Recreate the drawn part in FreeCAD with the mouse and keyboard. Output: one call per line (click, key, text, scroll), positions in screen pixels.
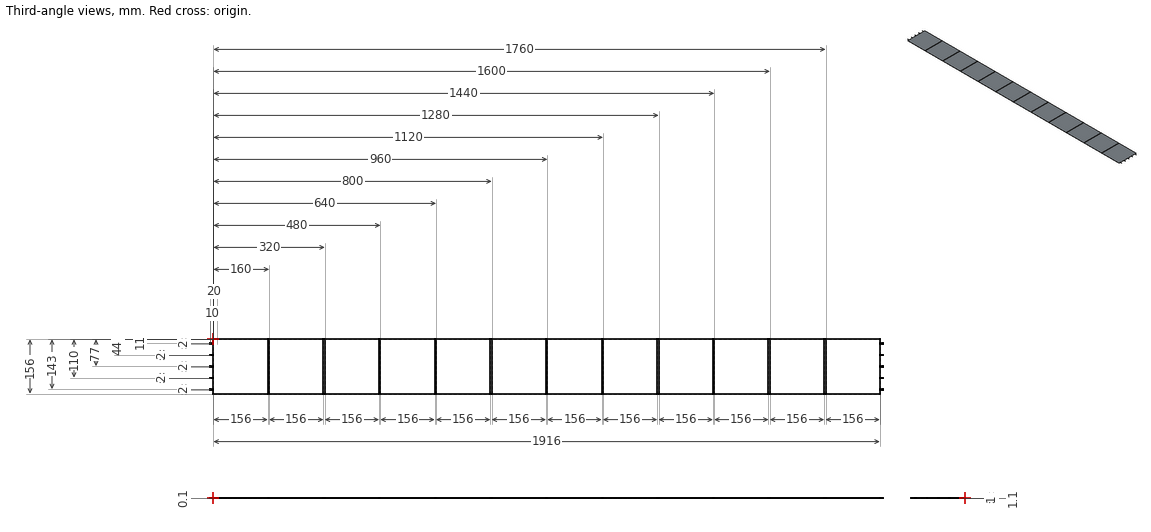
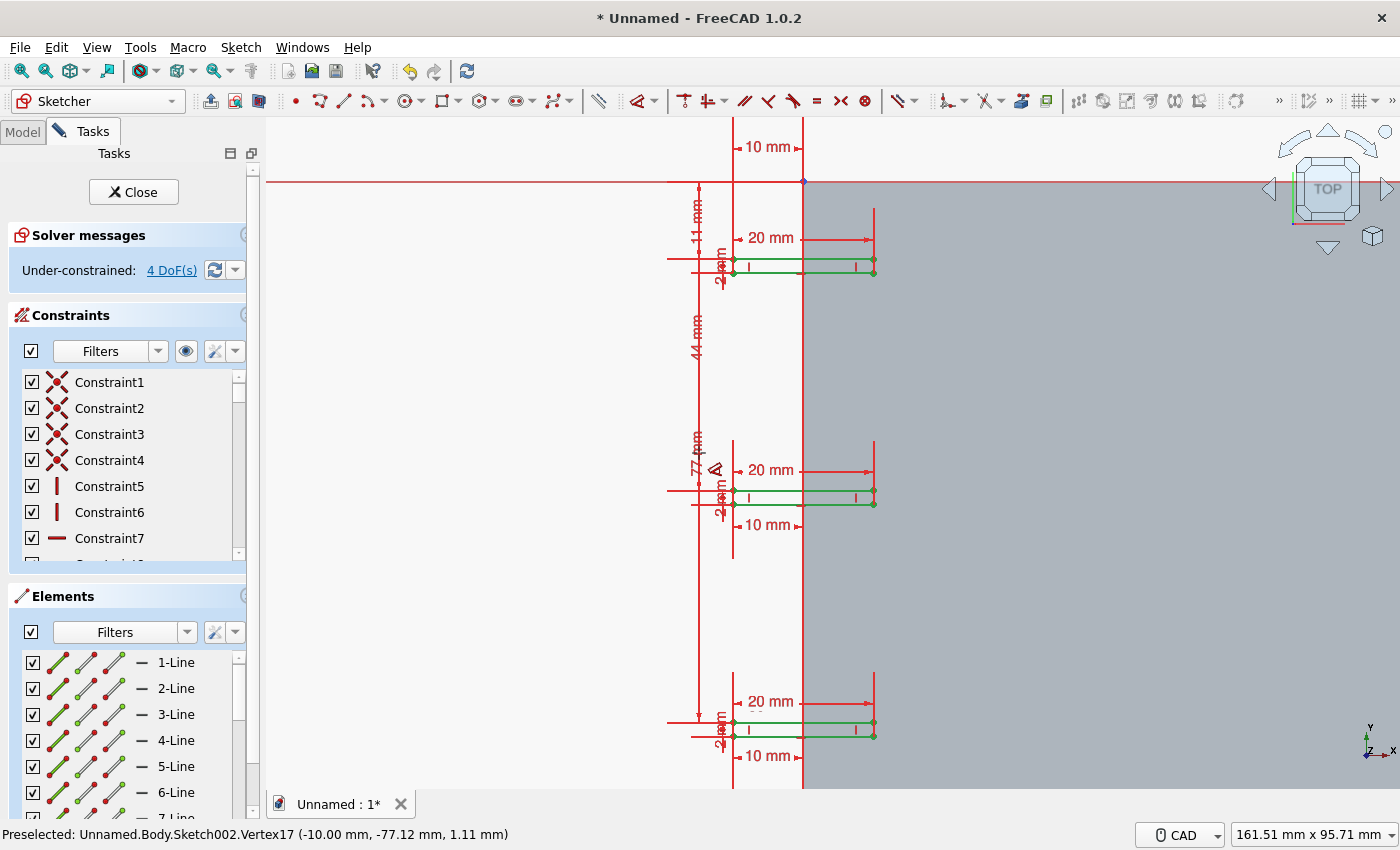
scroll(733, 259, down, 4)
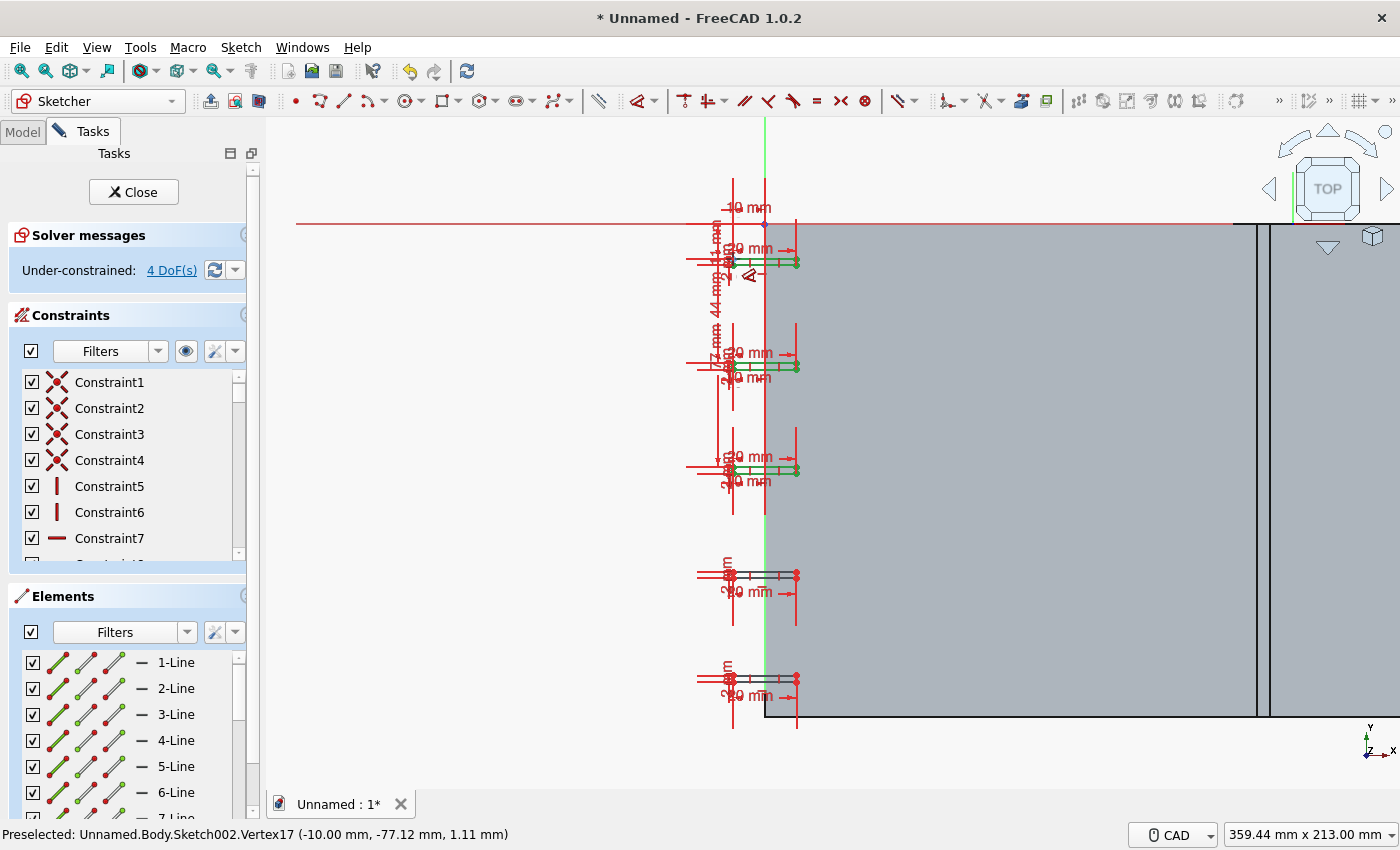
scroll(733, 572, up, 4)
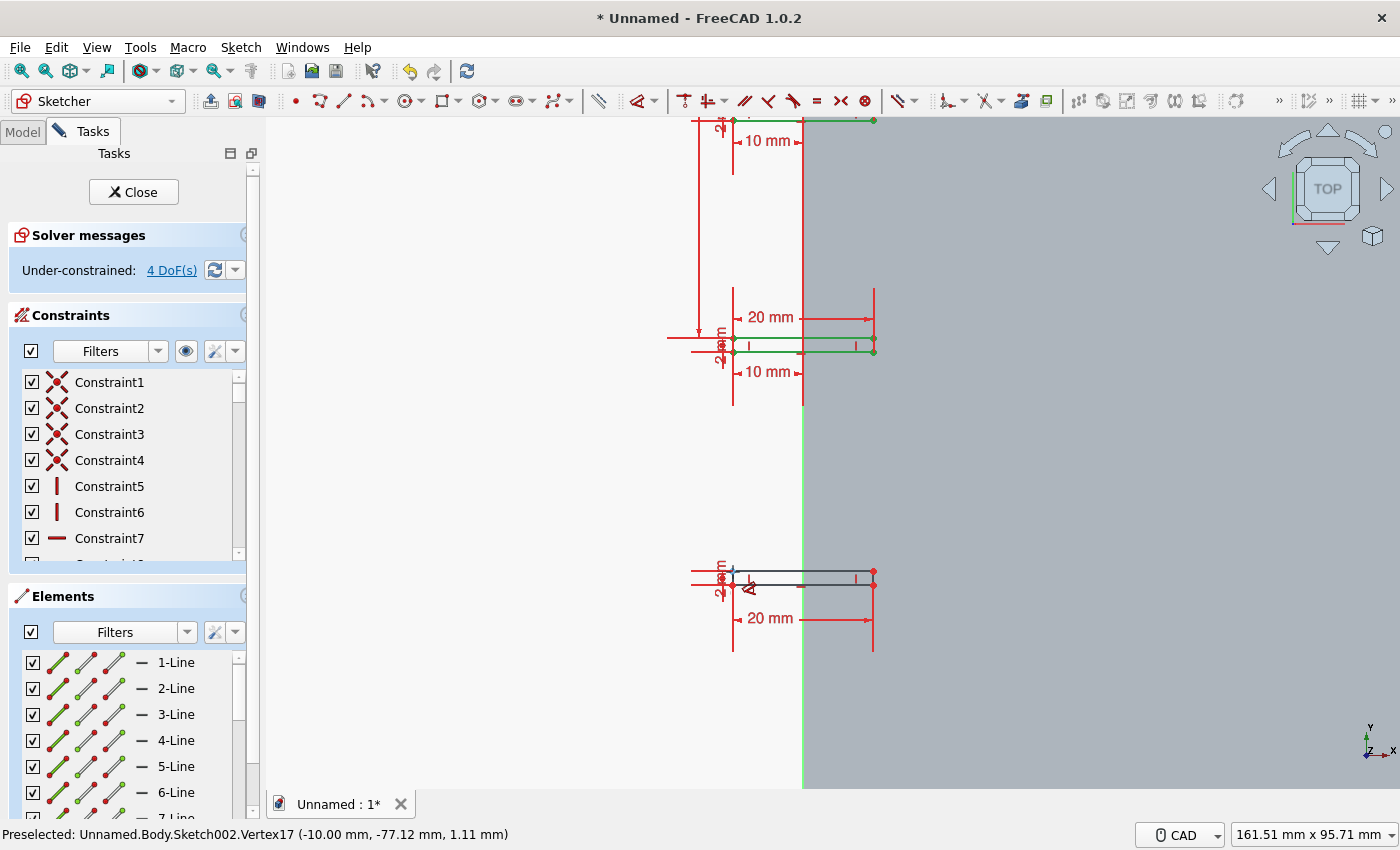
click(733, 571)
click(768, 653)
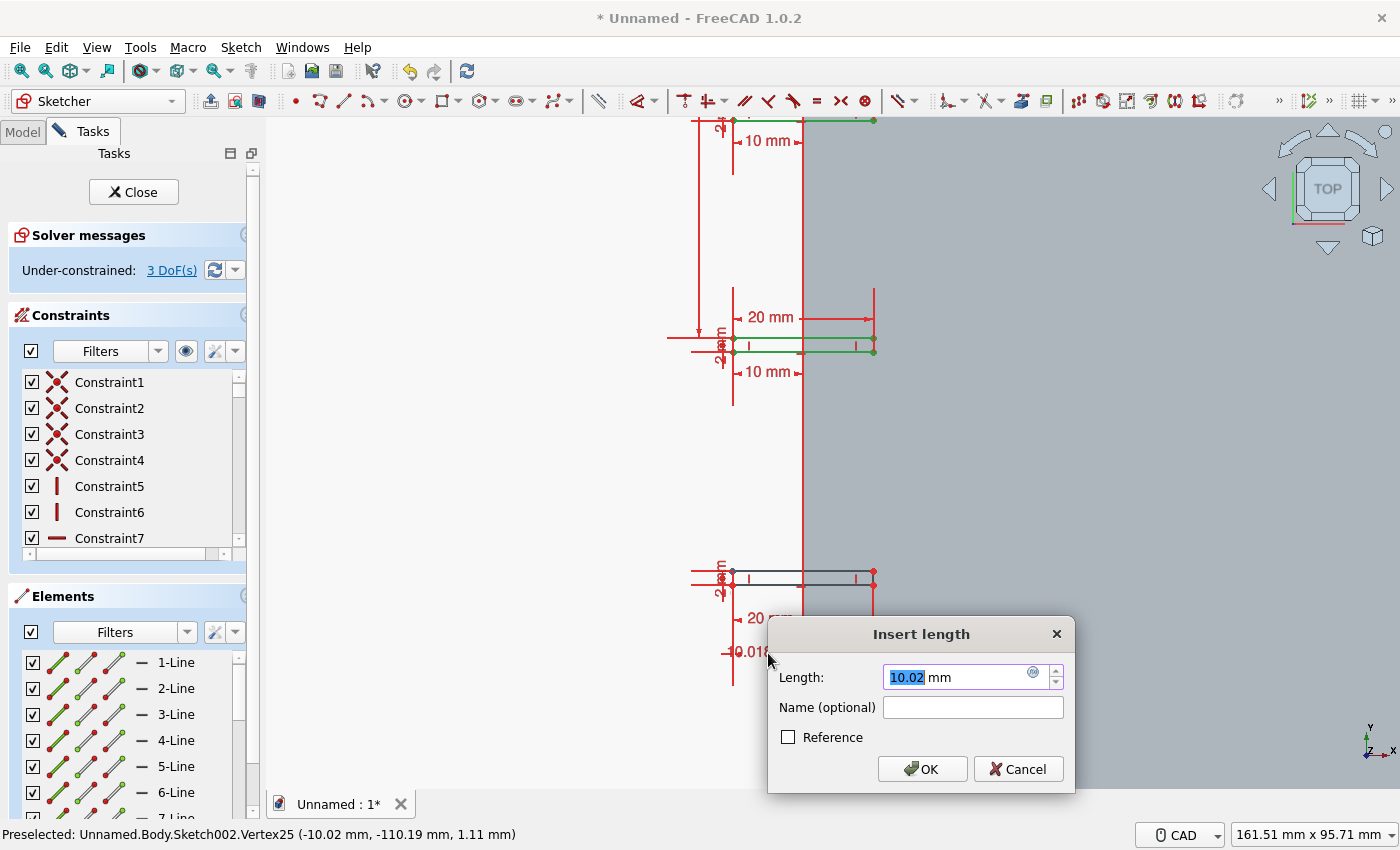
text(10)
key(Return)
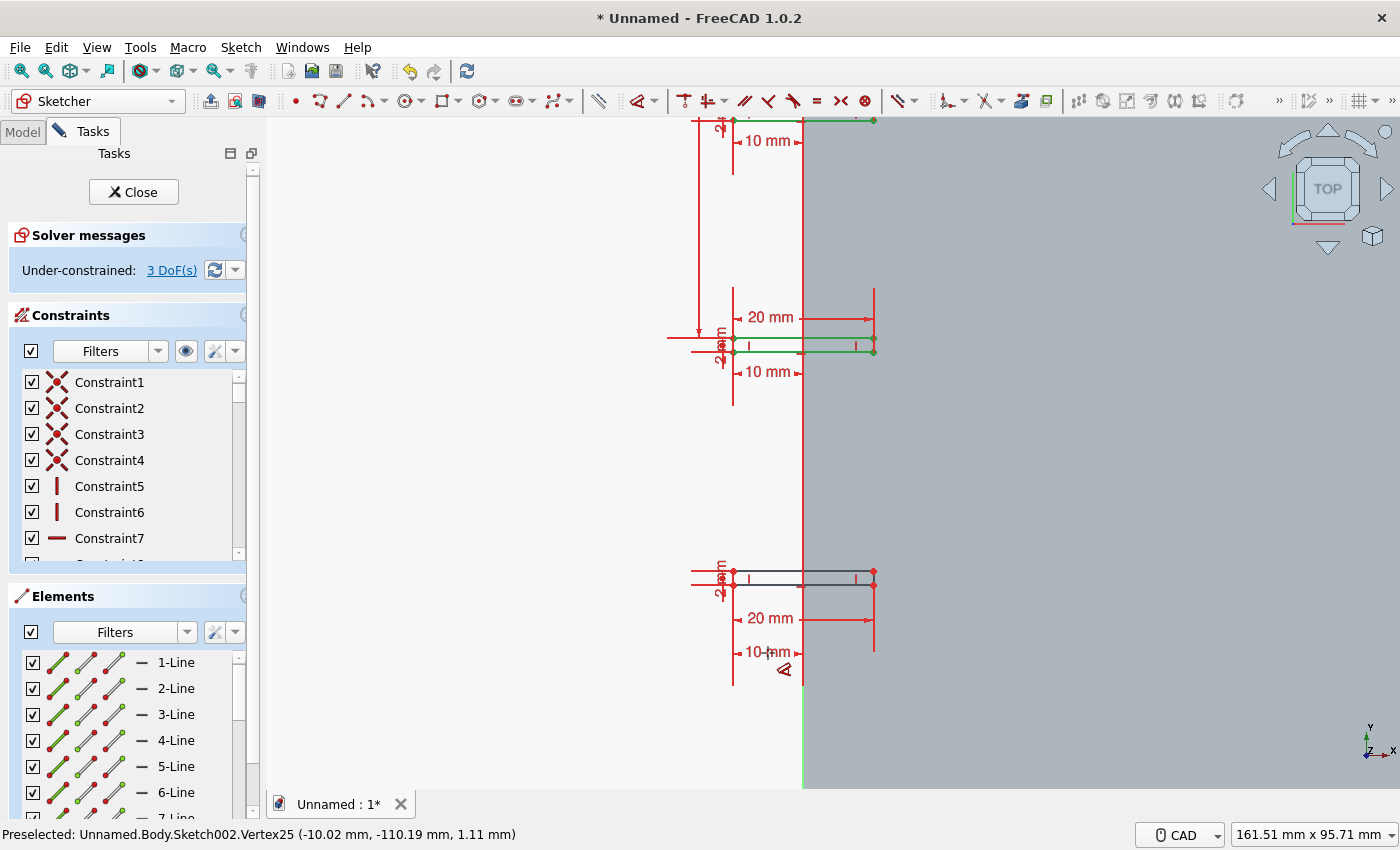
scroll(733, 572, down, 4)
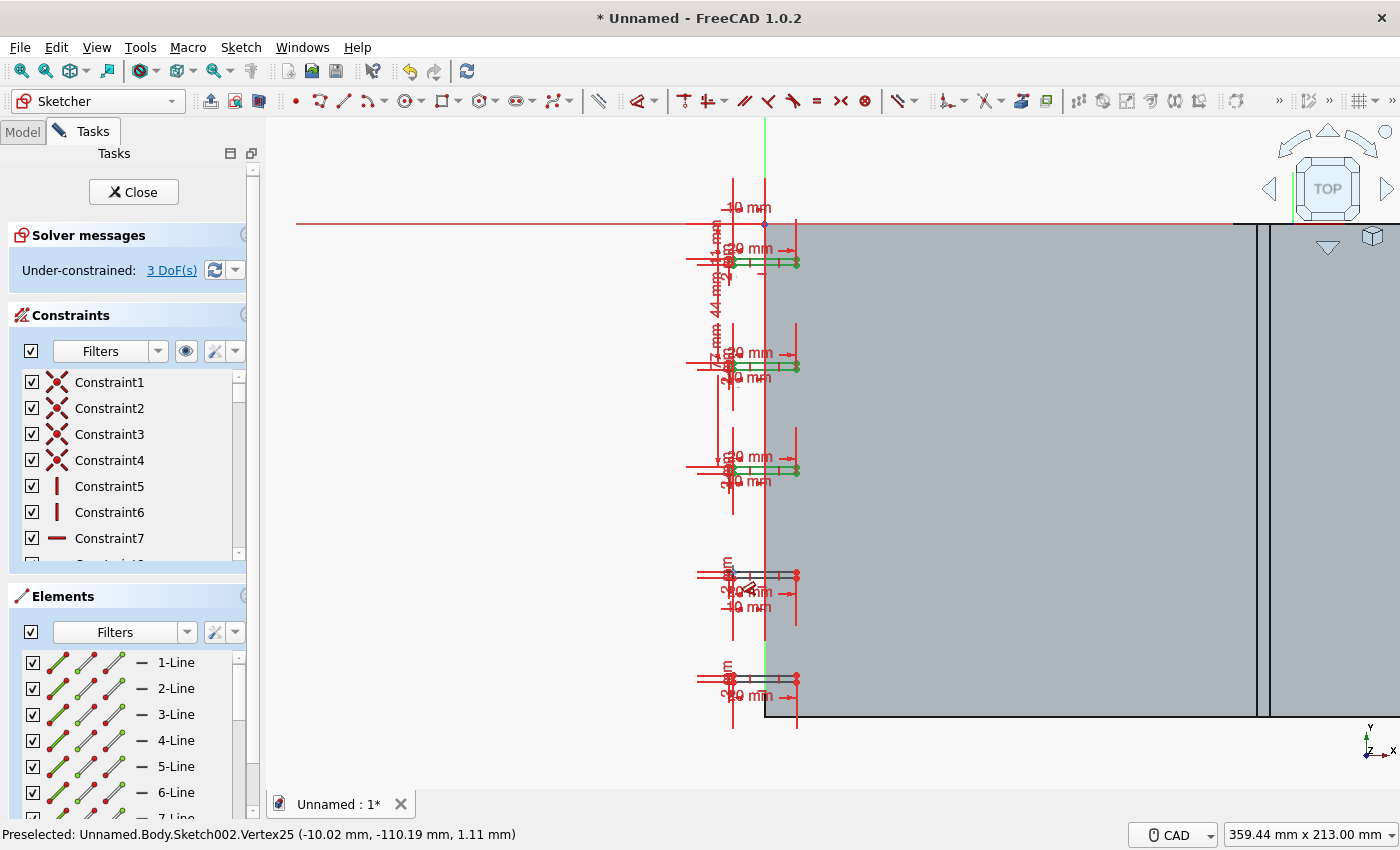
scroll(733, 676, up, 4)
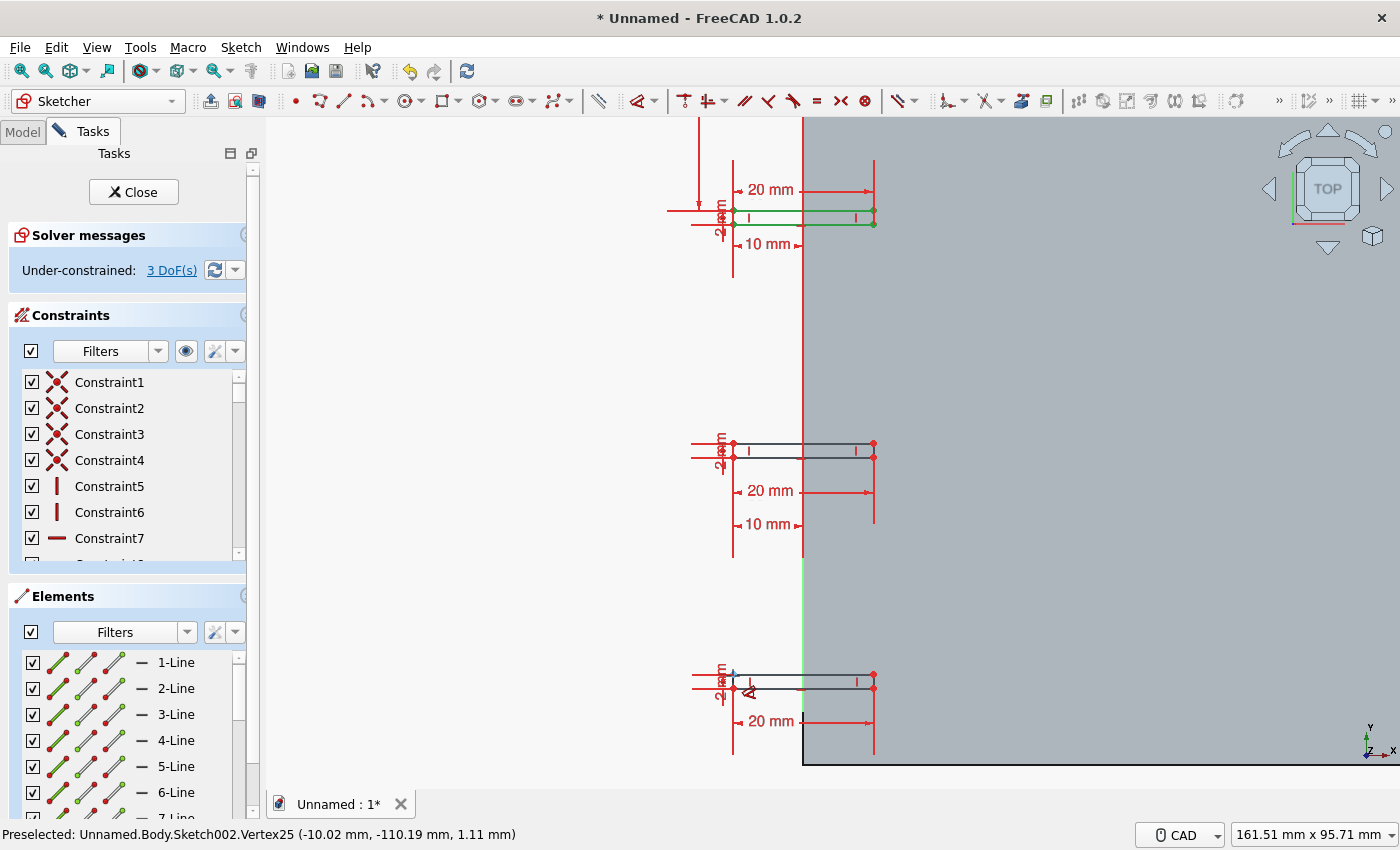
click(733, 675)
click(768, 757)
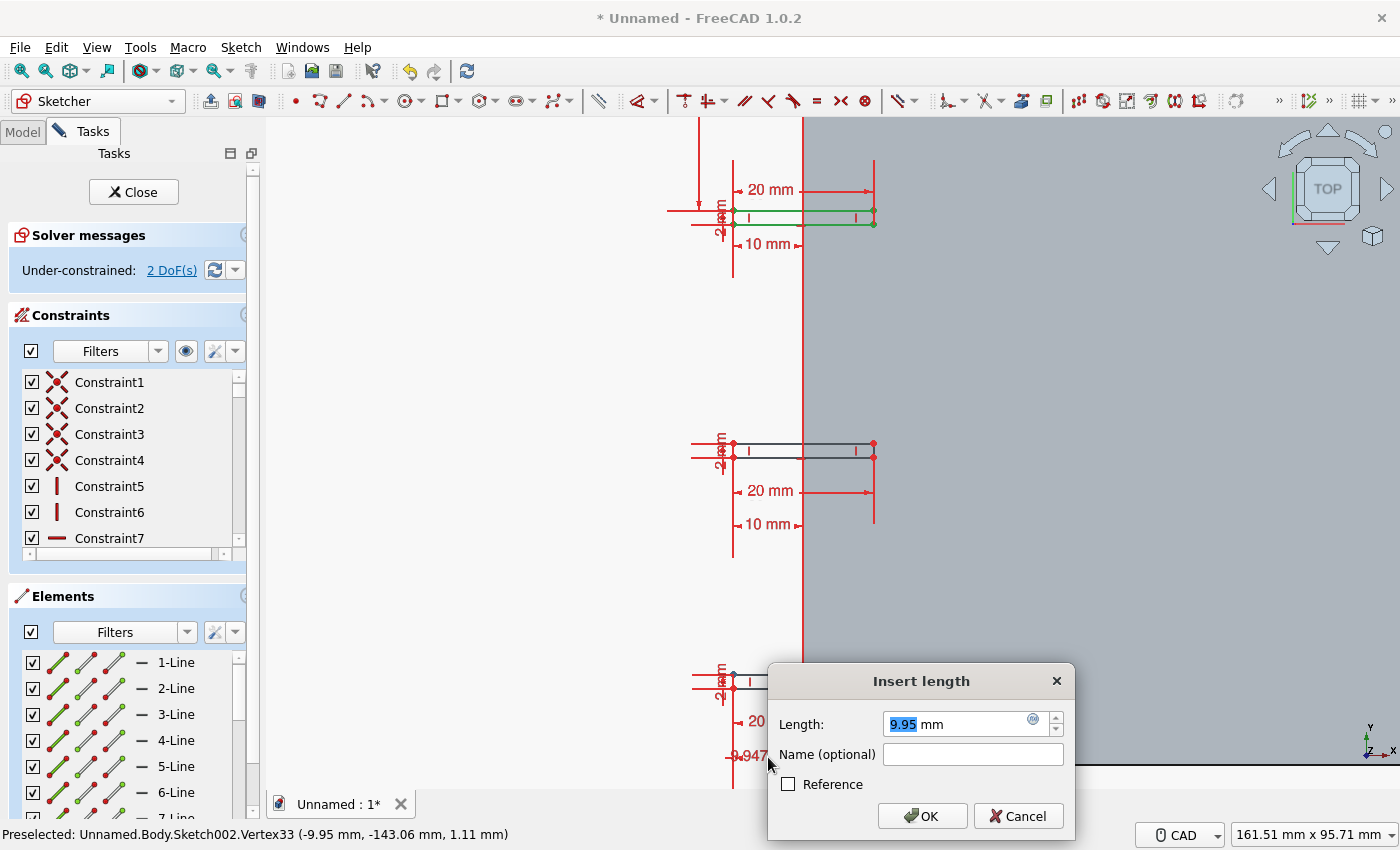
text(10)
key(Return)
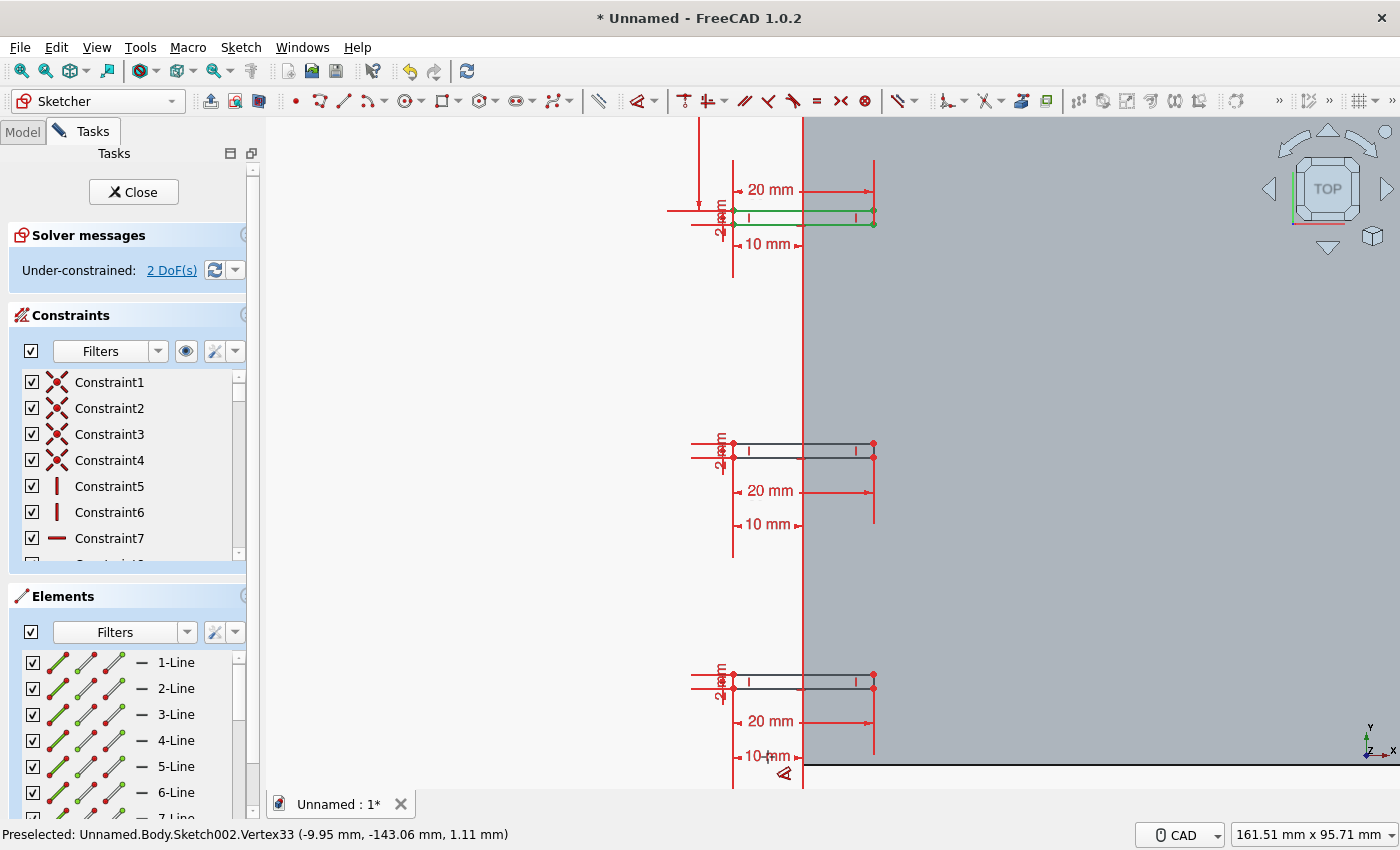
click(733, 444)
click(699, 294)